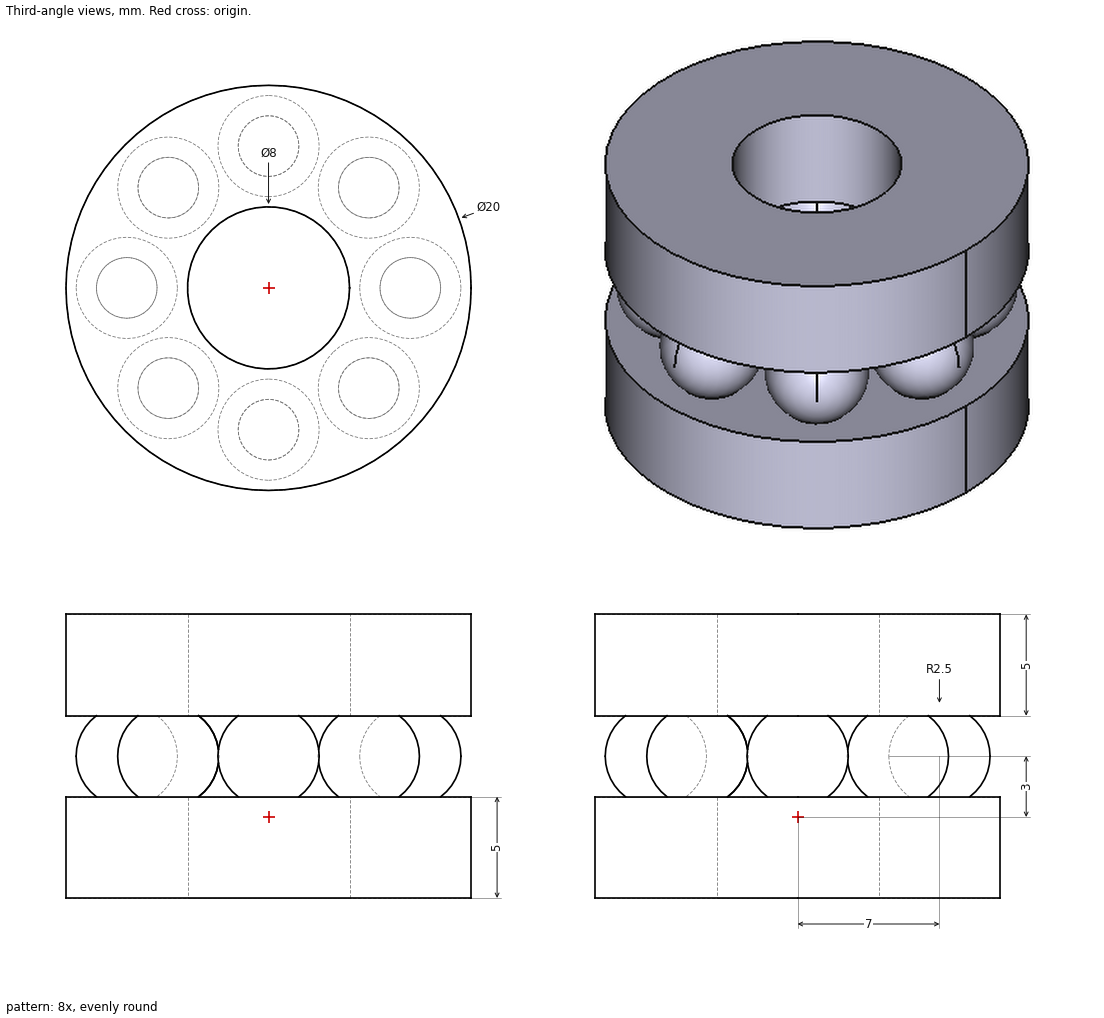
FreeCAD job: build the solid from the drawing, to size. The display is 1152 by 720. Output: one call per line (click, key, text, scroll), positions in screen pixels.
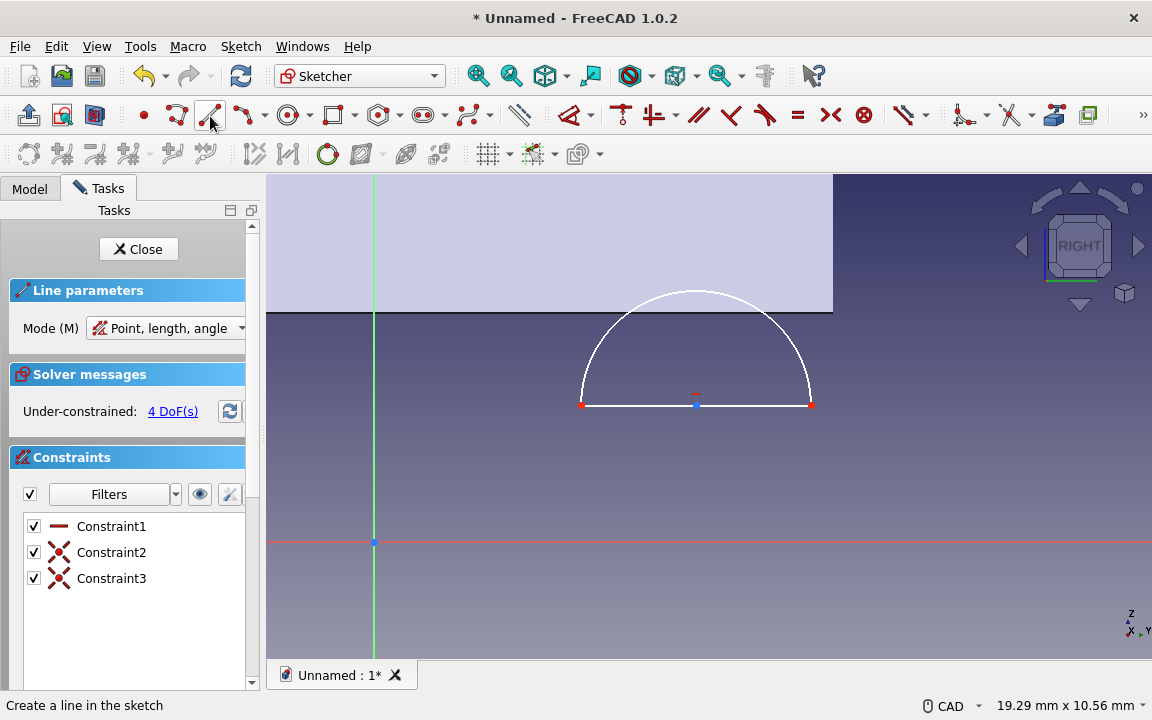
click(834, 405)
click(903, 405)
key(Escape)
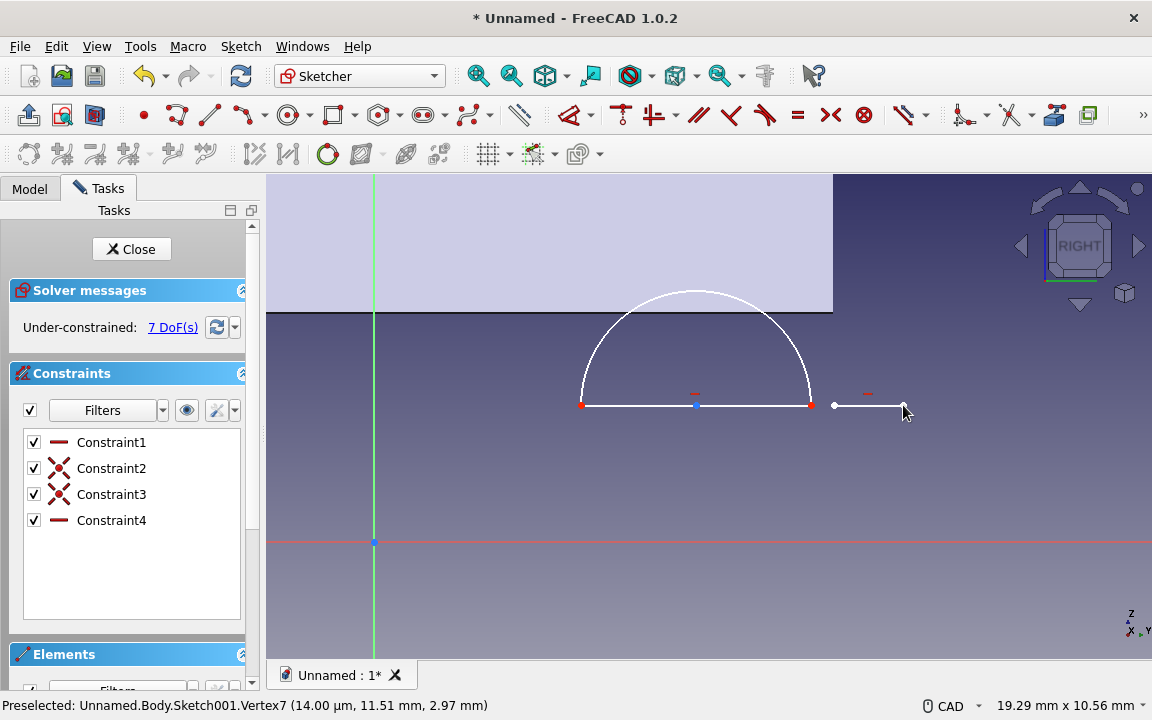
click(855, 406)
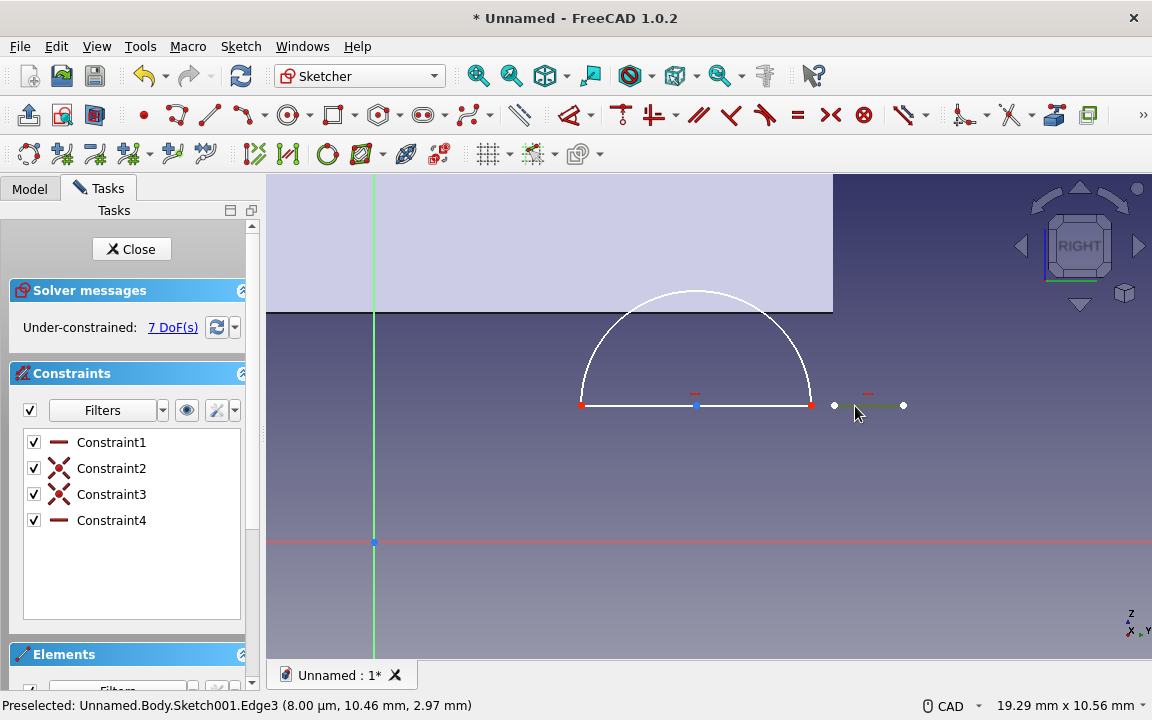
click(520, 116)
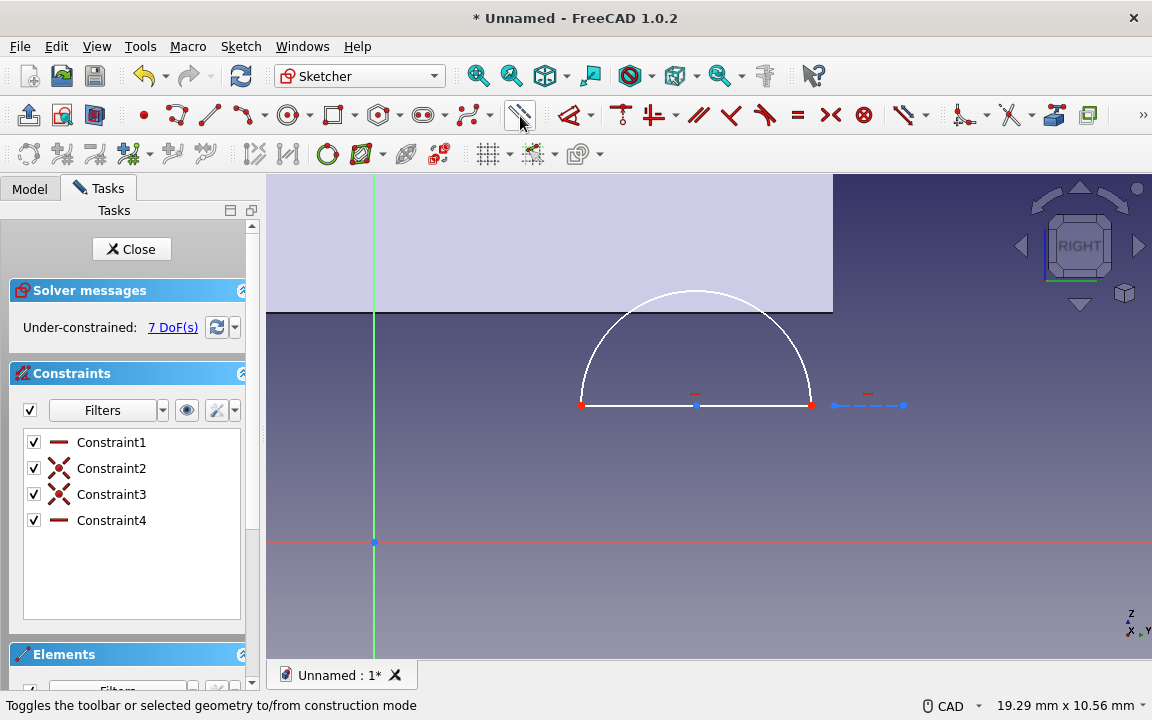
key(d)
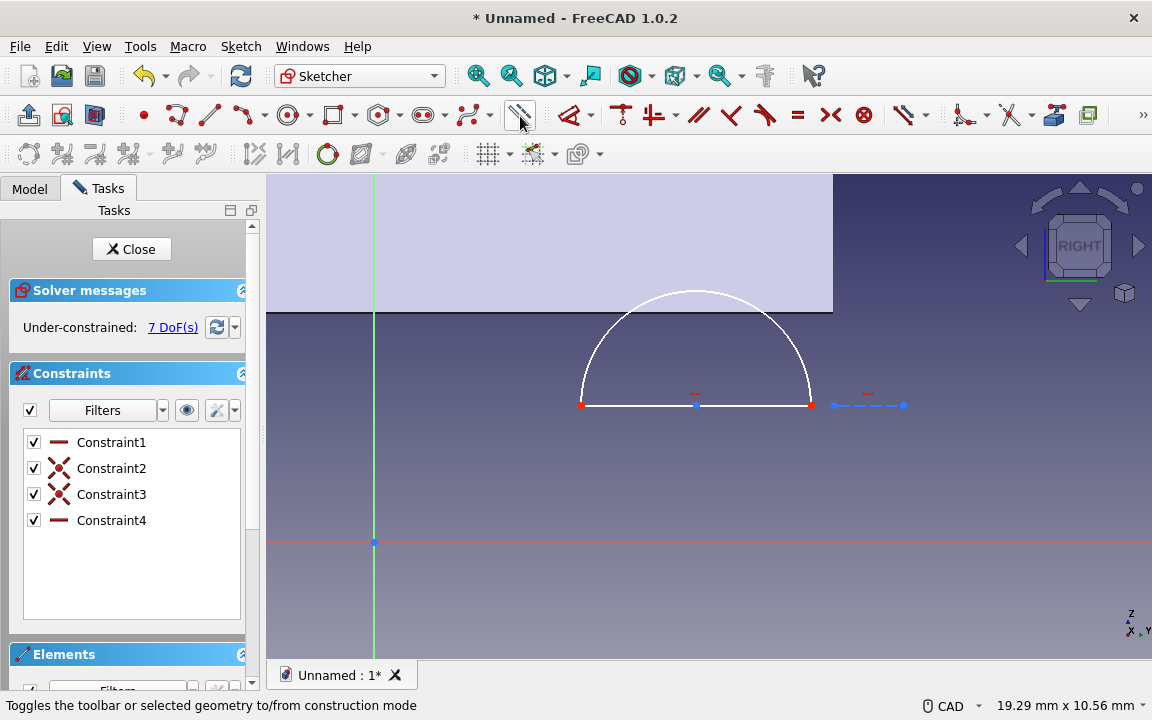
click(764, 313)
click(783, 287)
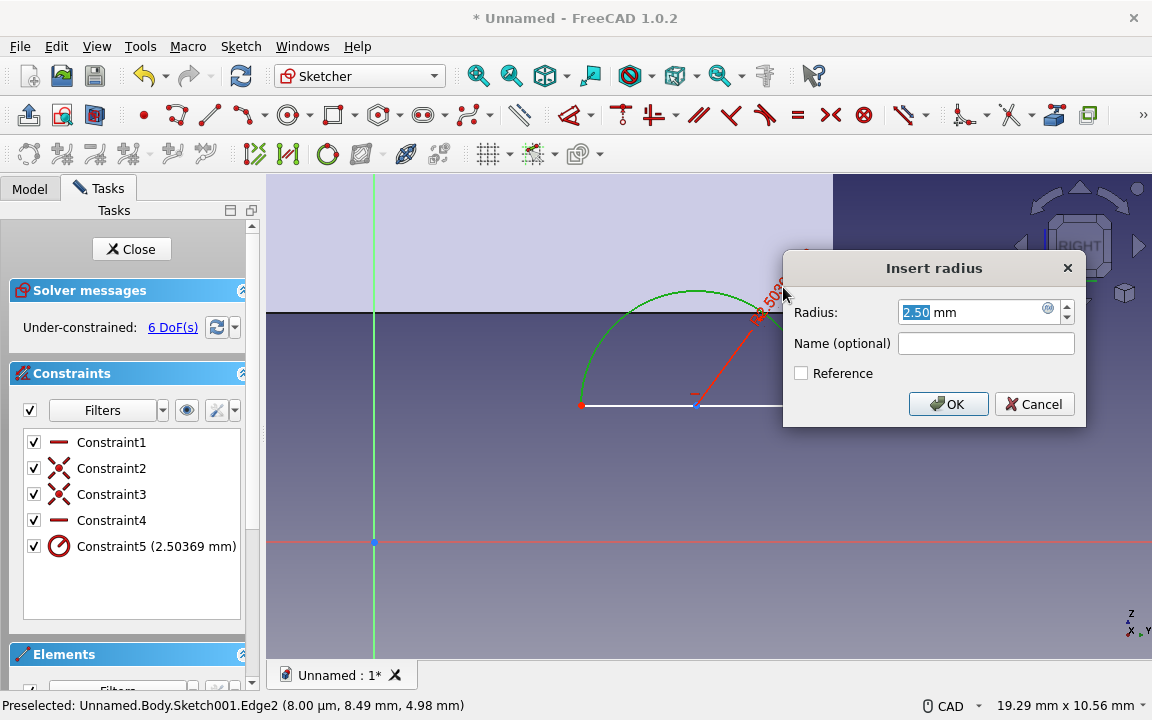
text(2.5)
key(Return)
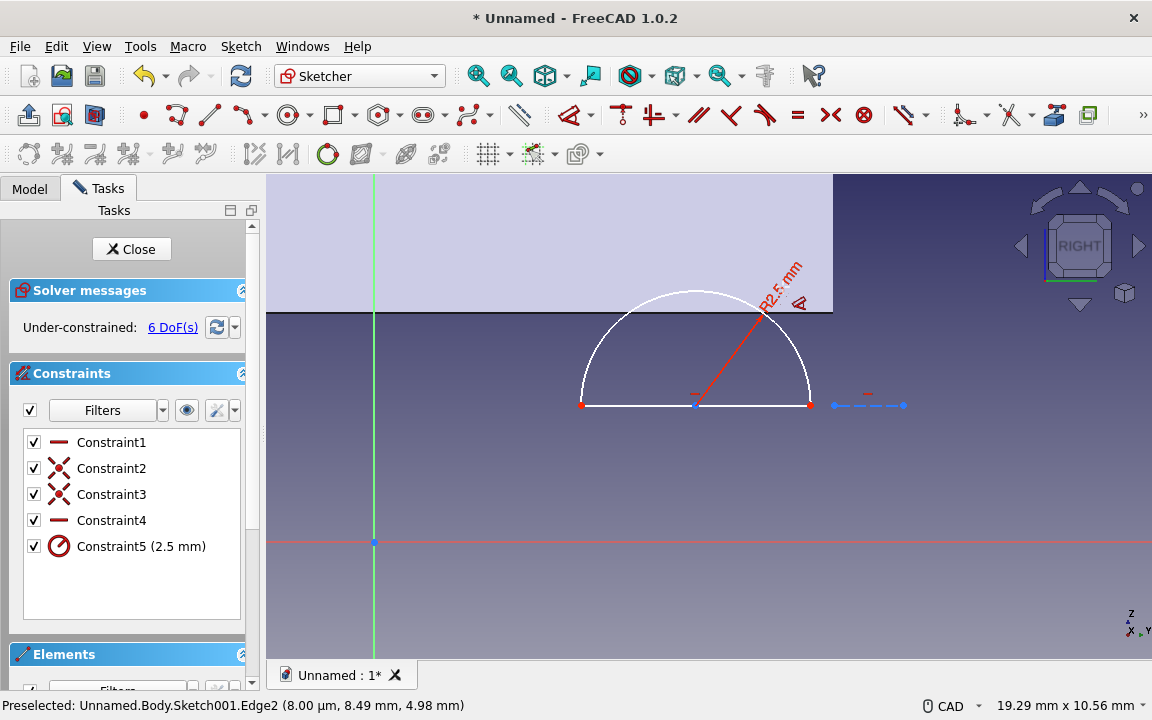
click(581, 406)
click(340, 474)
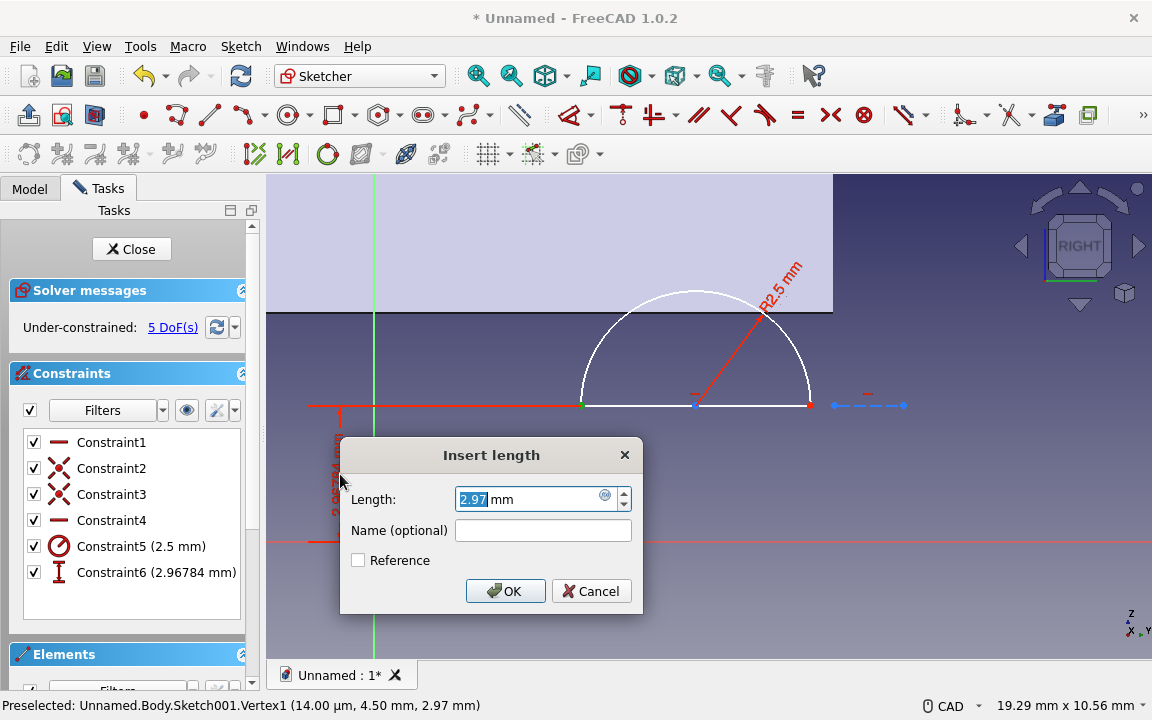
text(3)
key(Return)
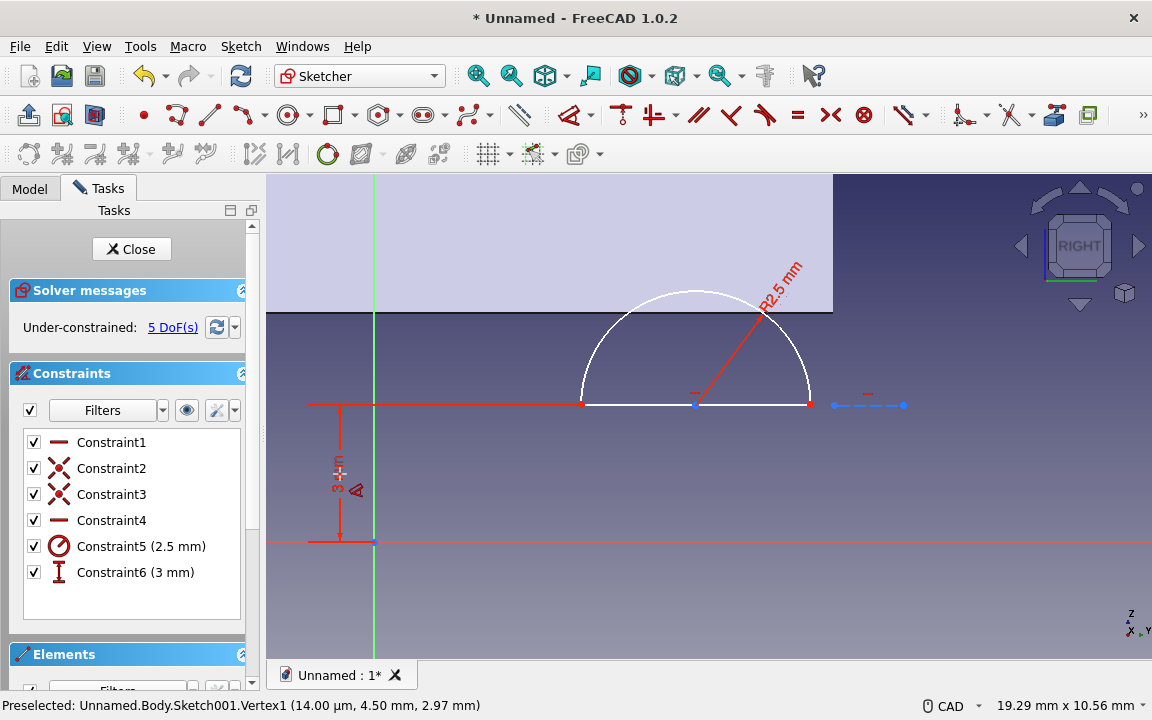
click(834, 406)
click(340, 443)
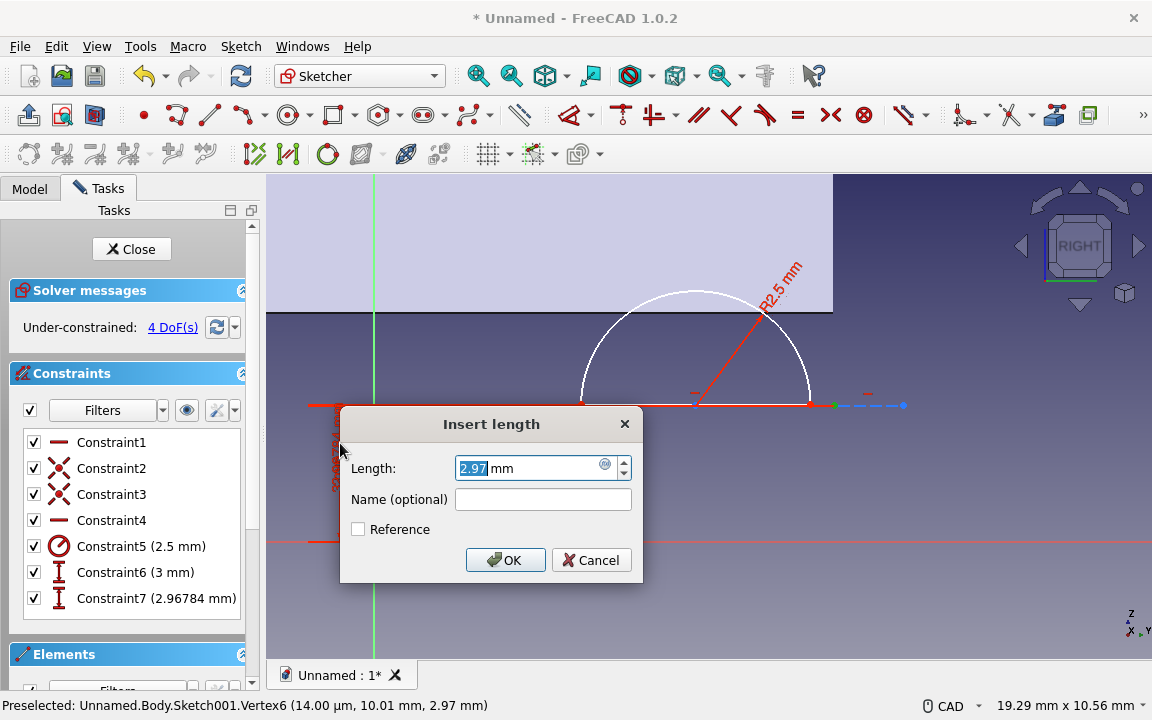
text(3)
key(Return)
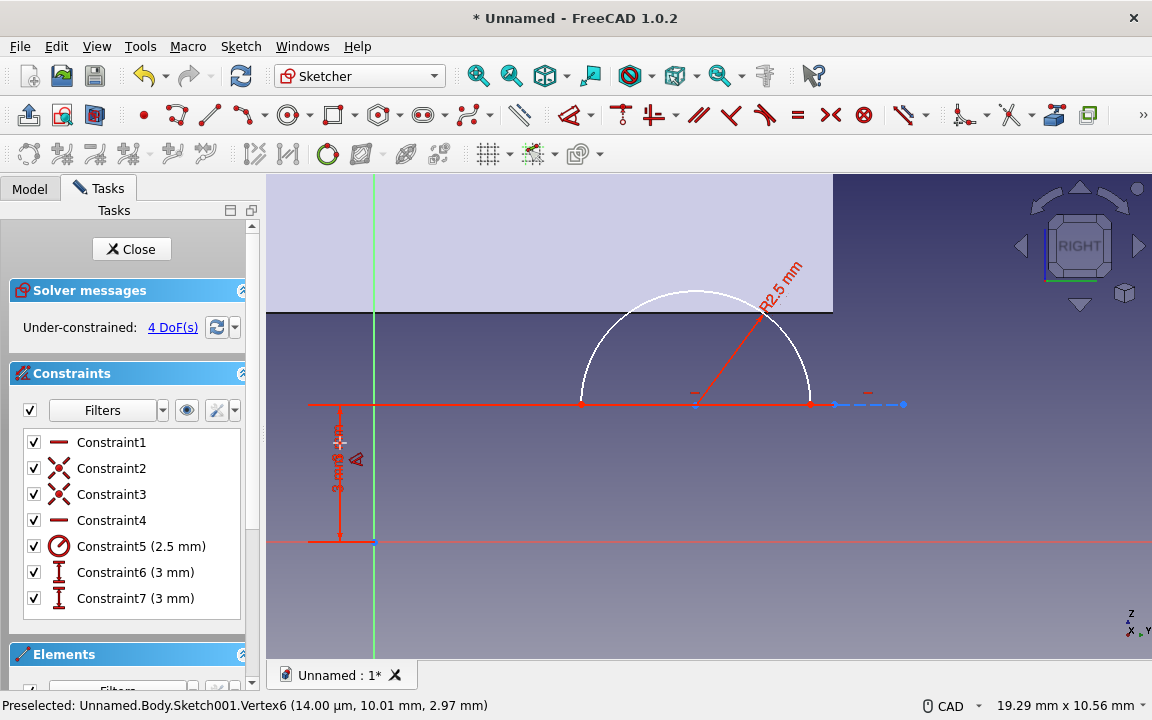
click(696, 406)
click(535, 576)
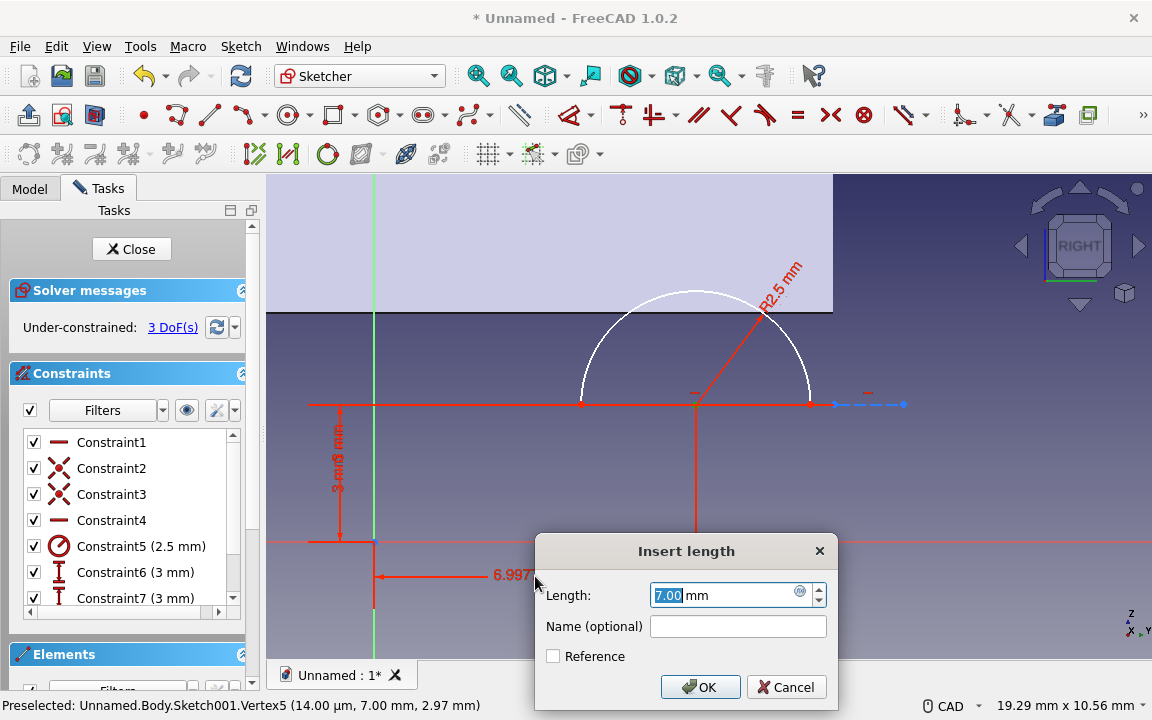
text(7)
key(Return)